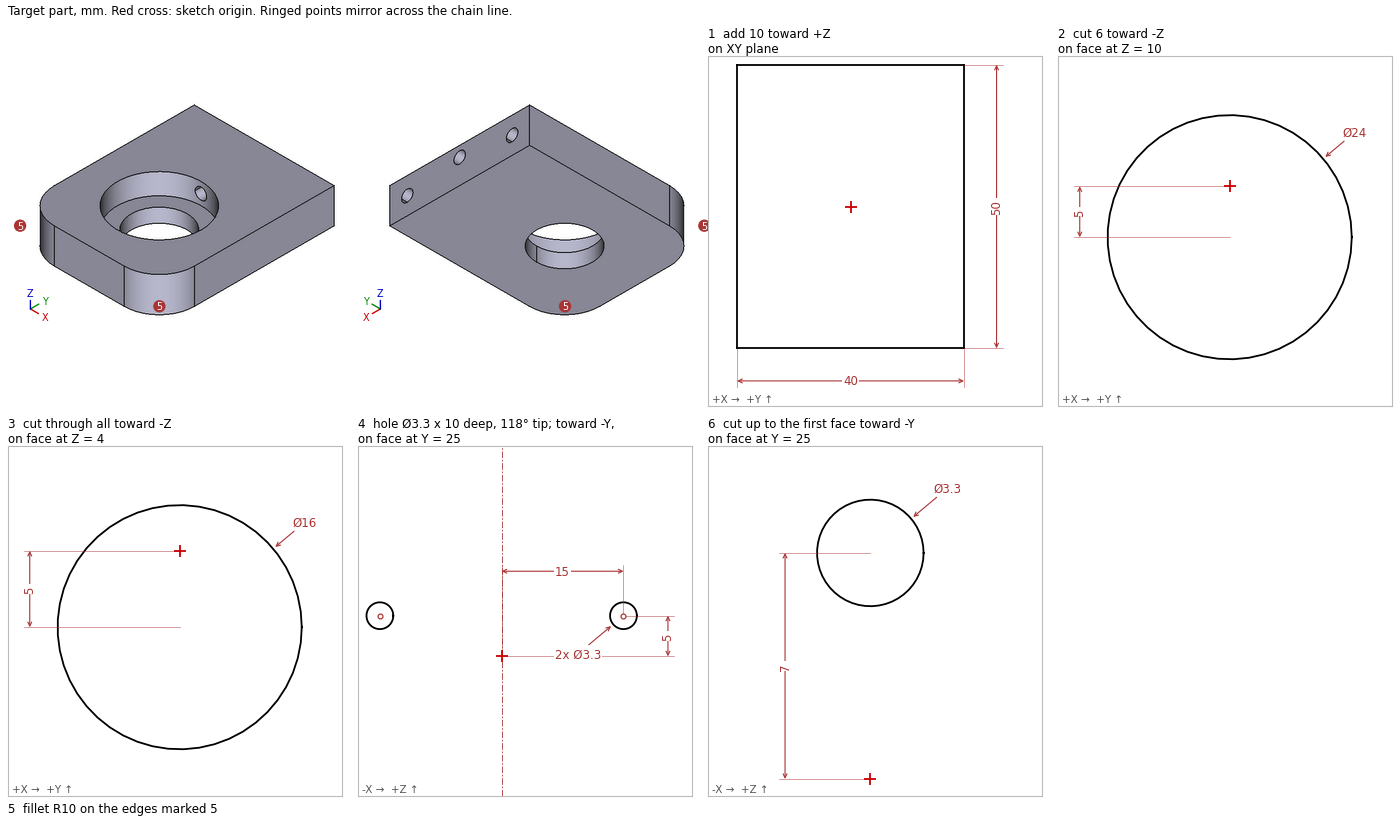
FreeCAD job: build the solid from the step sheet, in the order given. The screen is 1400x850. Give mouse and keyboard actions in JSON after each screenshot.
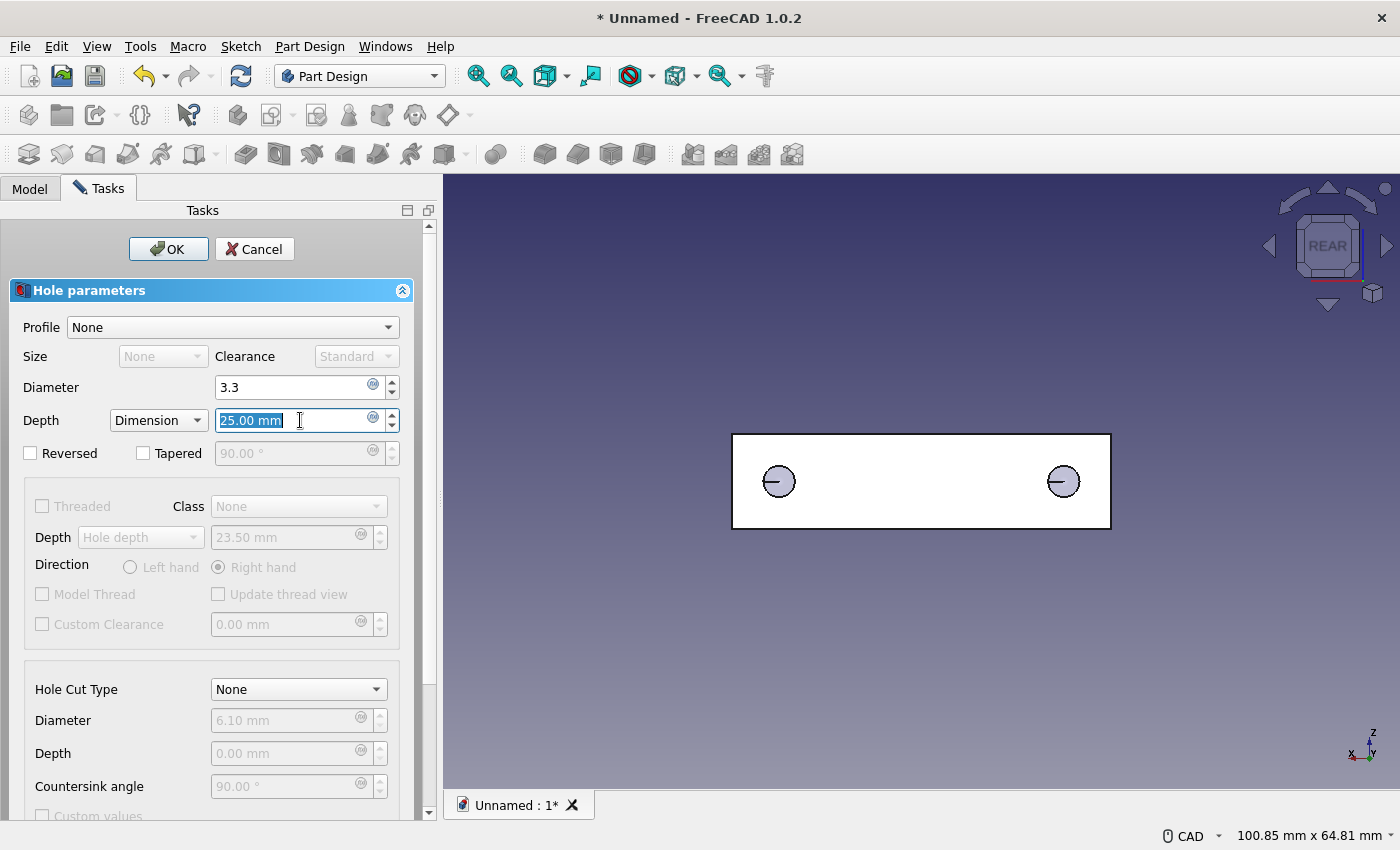
{"action": "type", "text": "10"}
{"action": "key", "text": "Tab"}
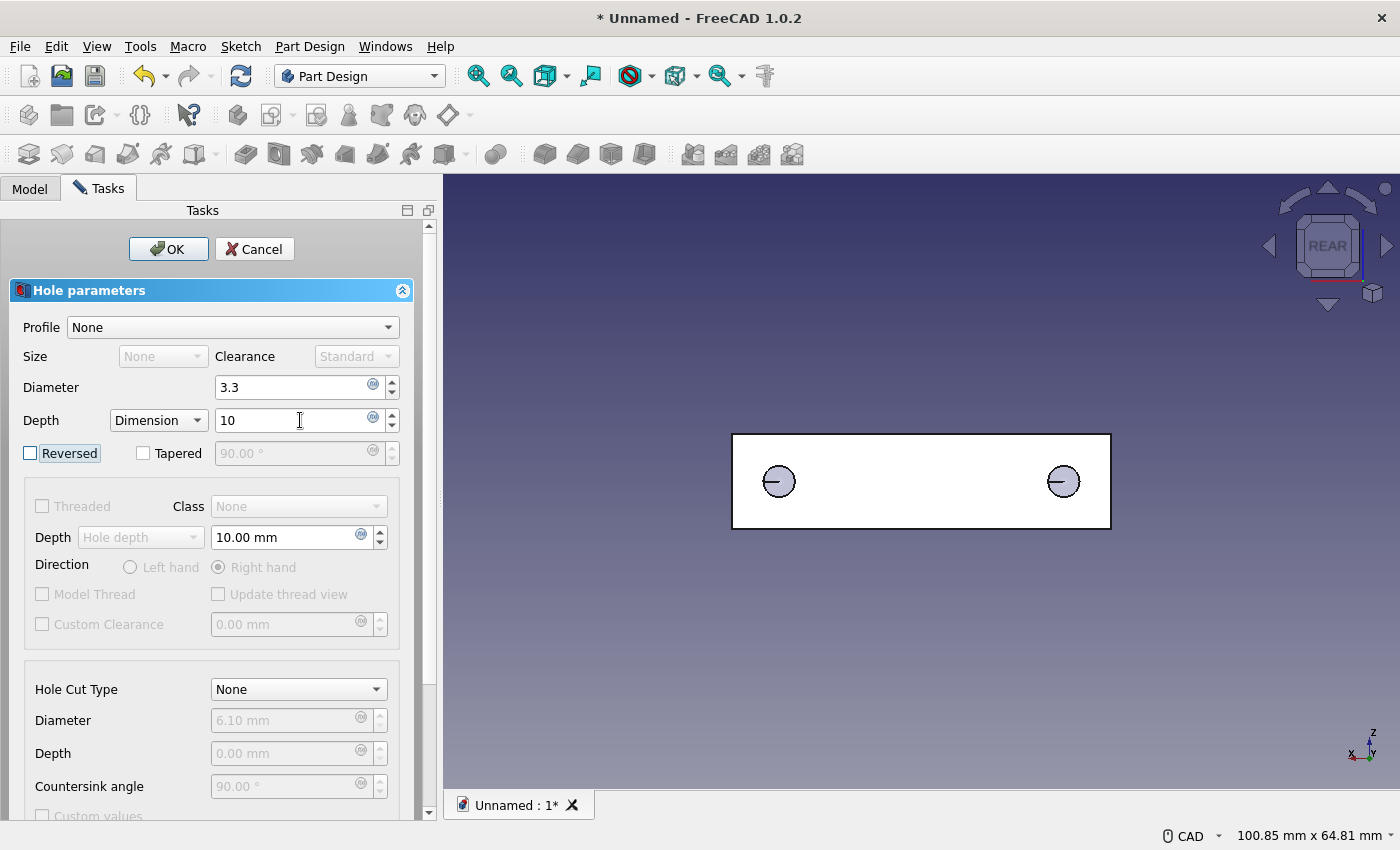
{"action": "left_click", "coordinate": [169, 249]}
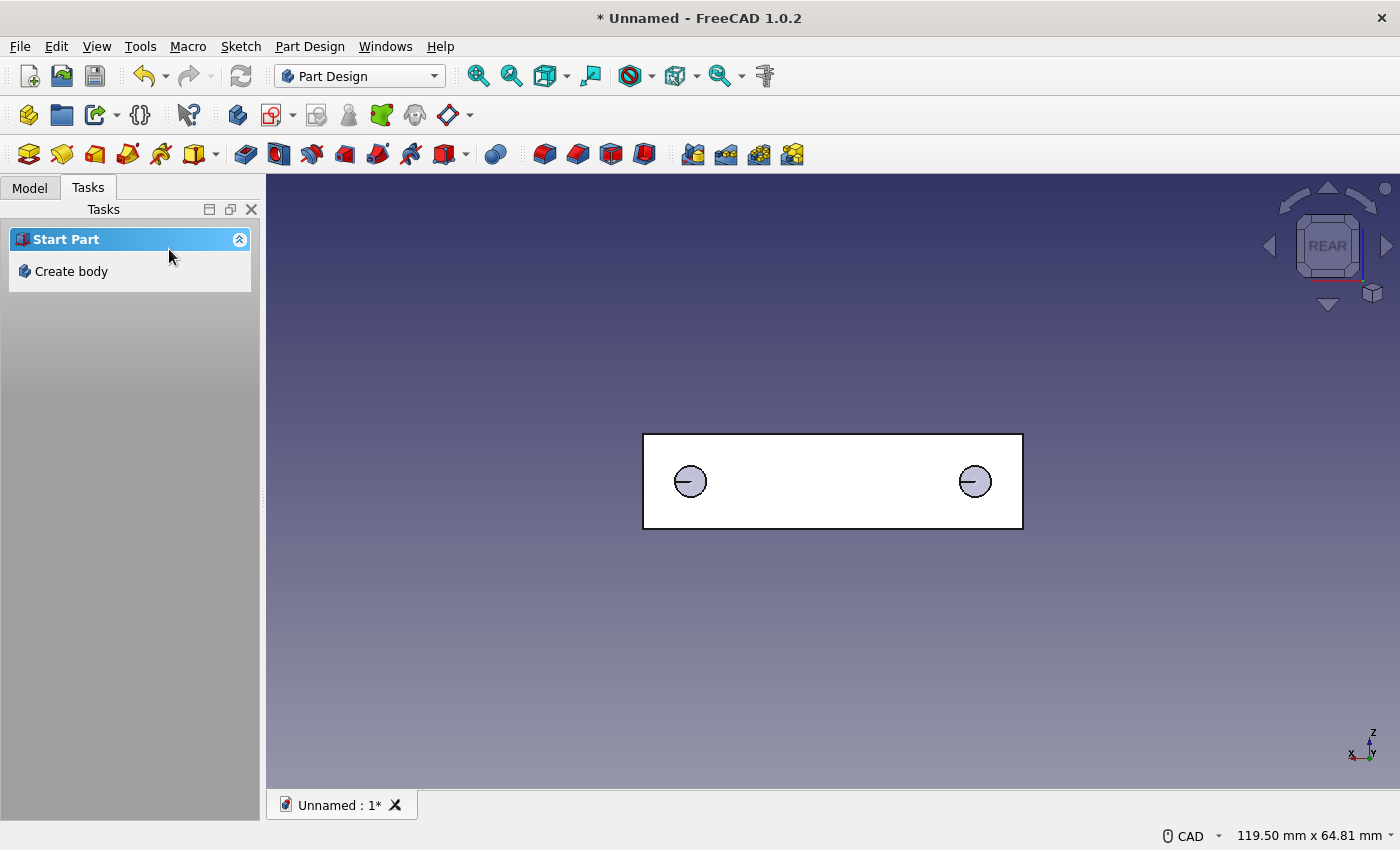
{"action": "left_click", "coordinate": [479, 76]}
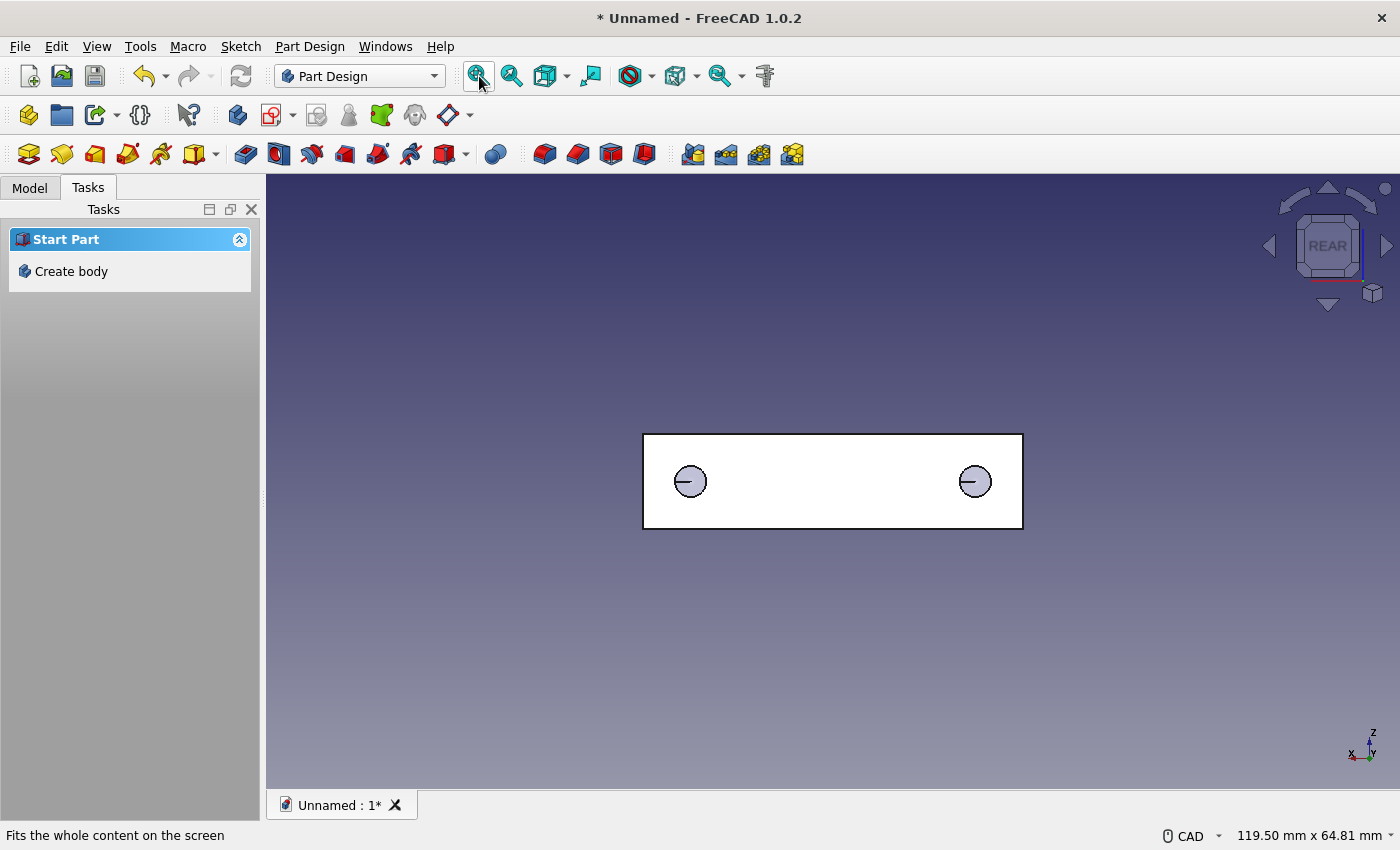
{"action": "key", "text": "0"}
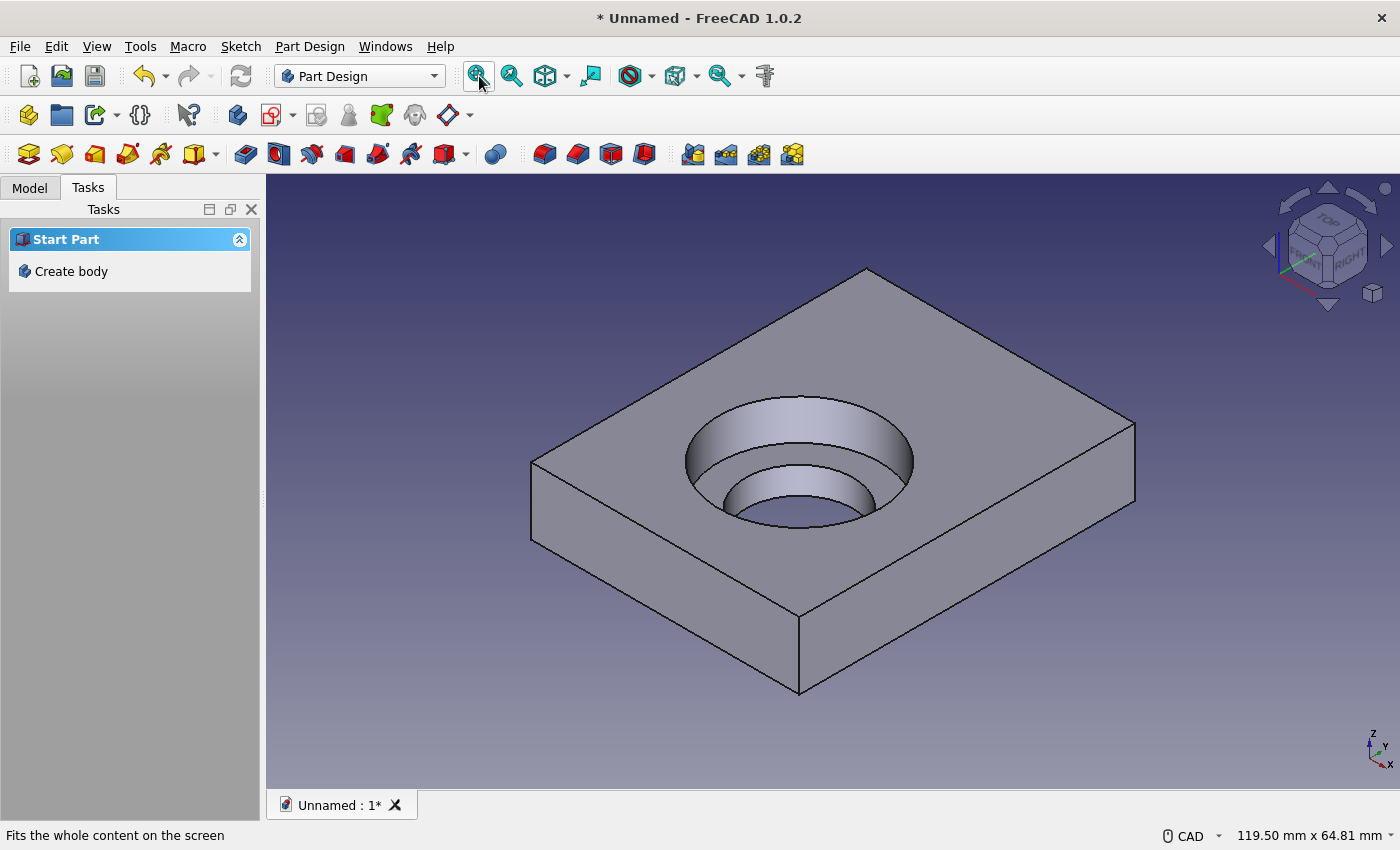
{"action": "left_click", "coordinate": [799, 655]}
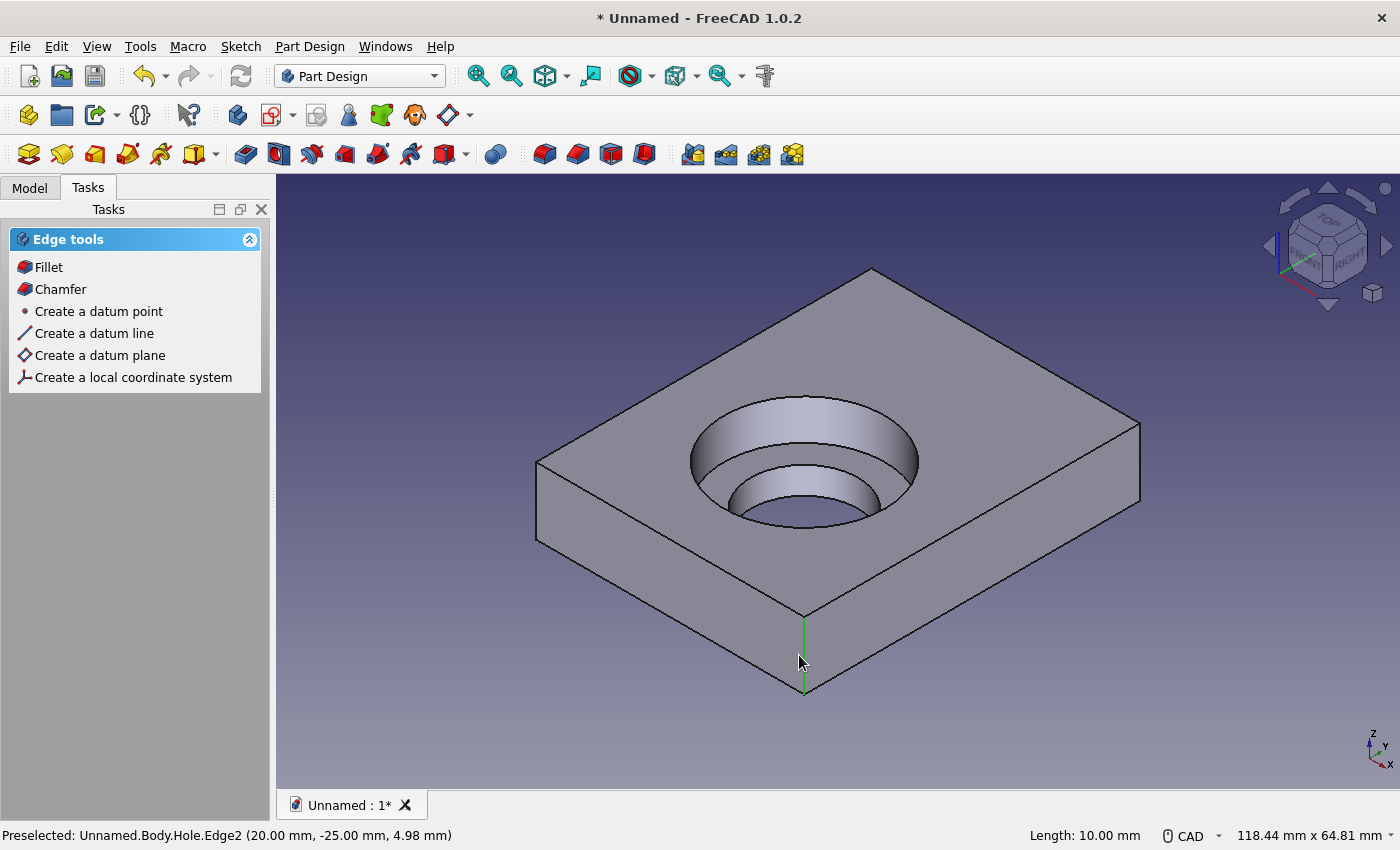
{"action": "key", "text": "2"}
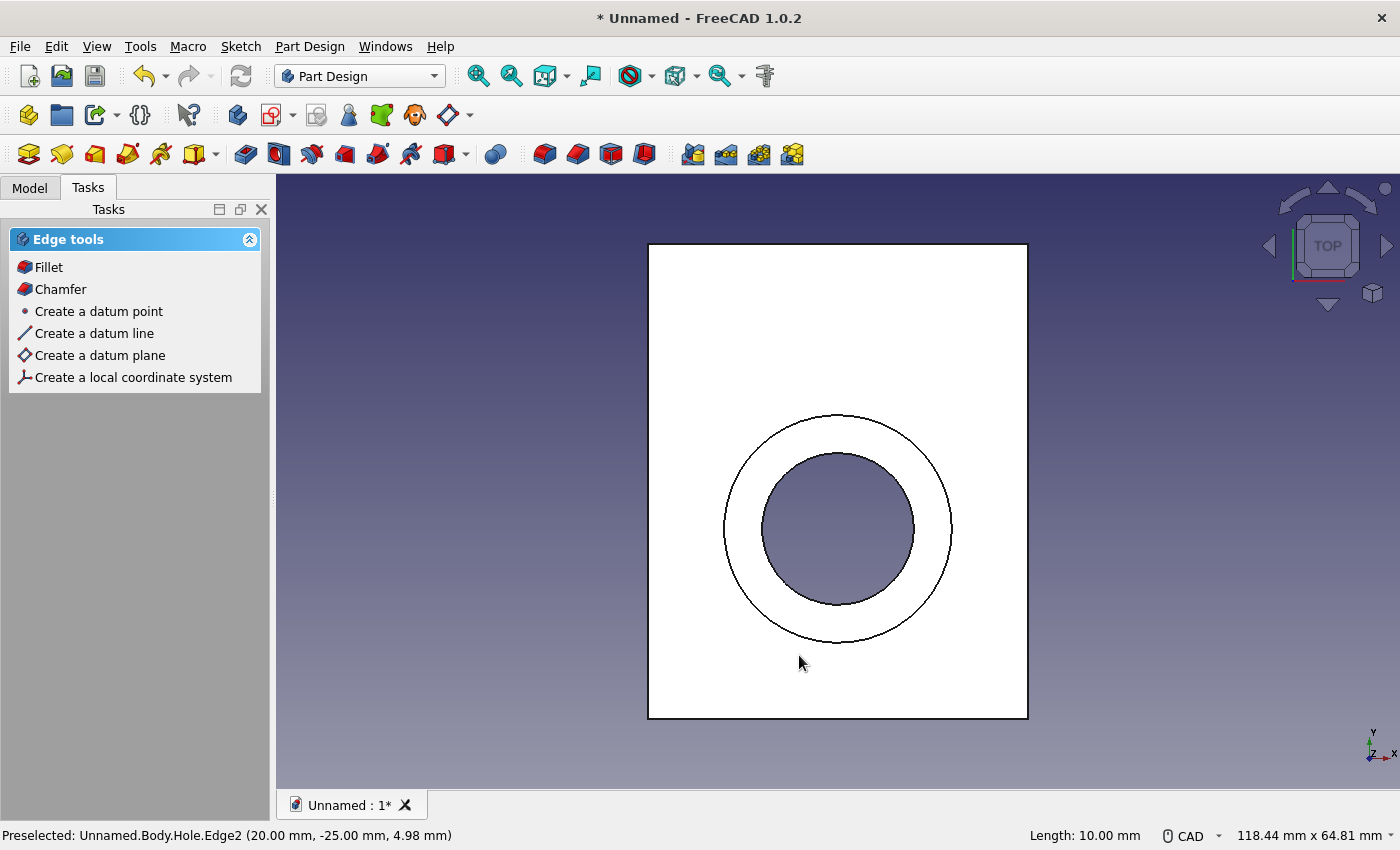
{"action": "key", "text": "1"}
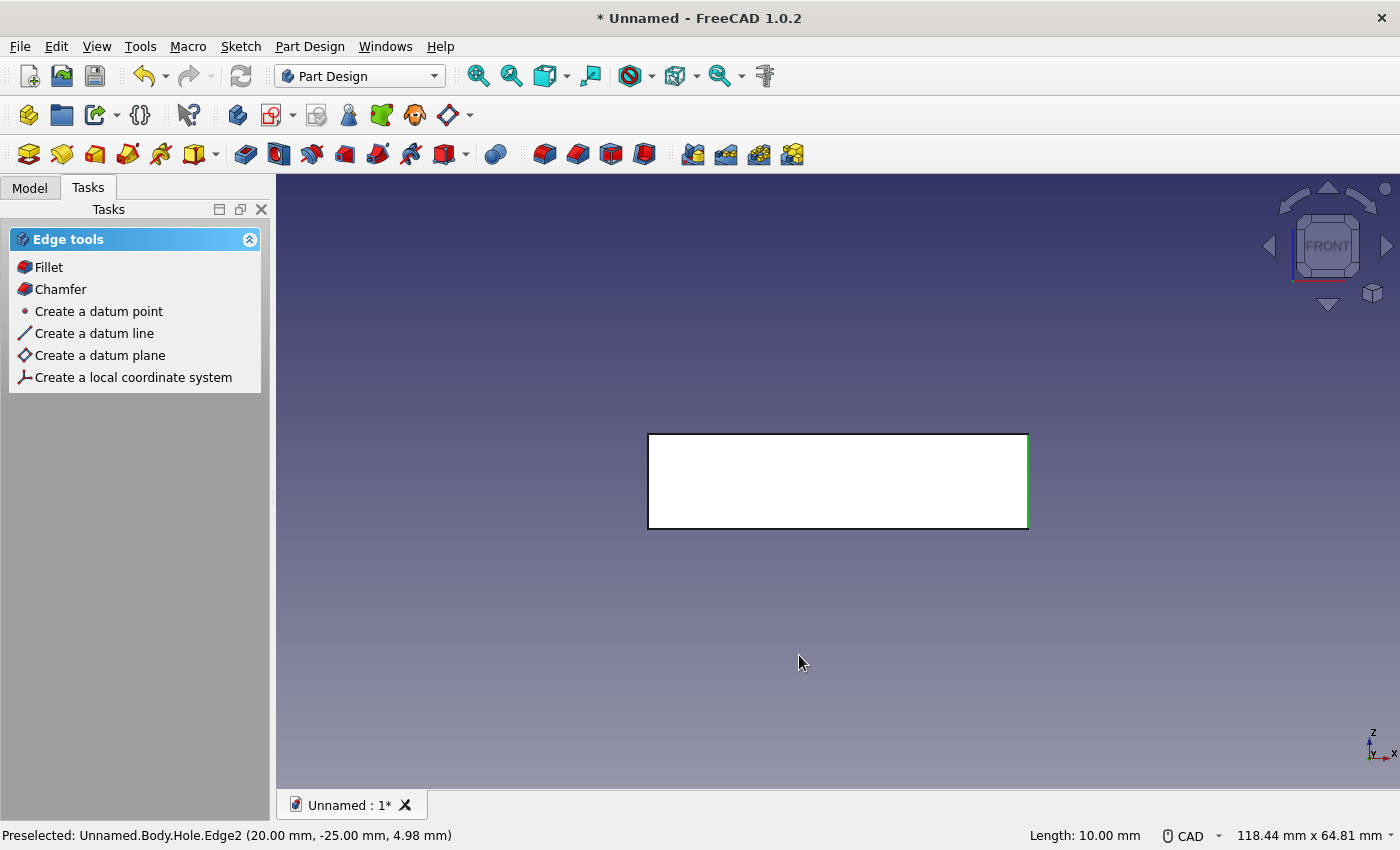
{"action": "left_click", "coordinate": [479, 76]}